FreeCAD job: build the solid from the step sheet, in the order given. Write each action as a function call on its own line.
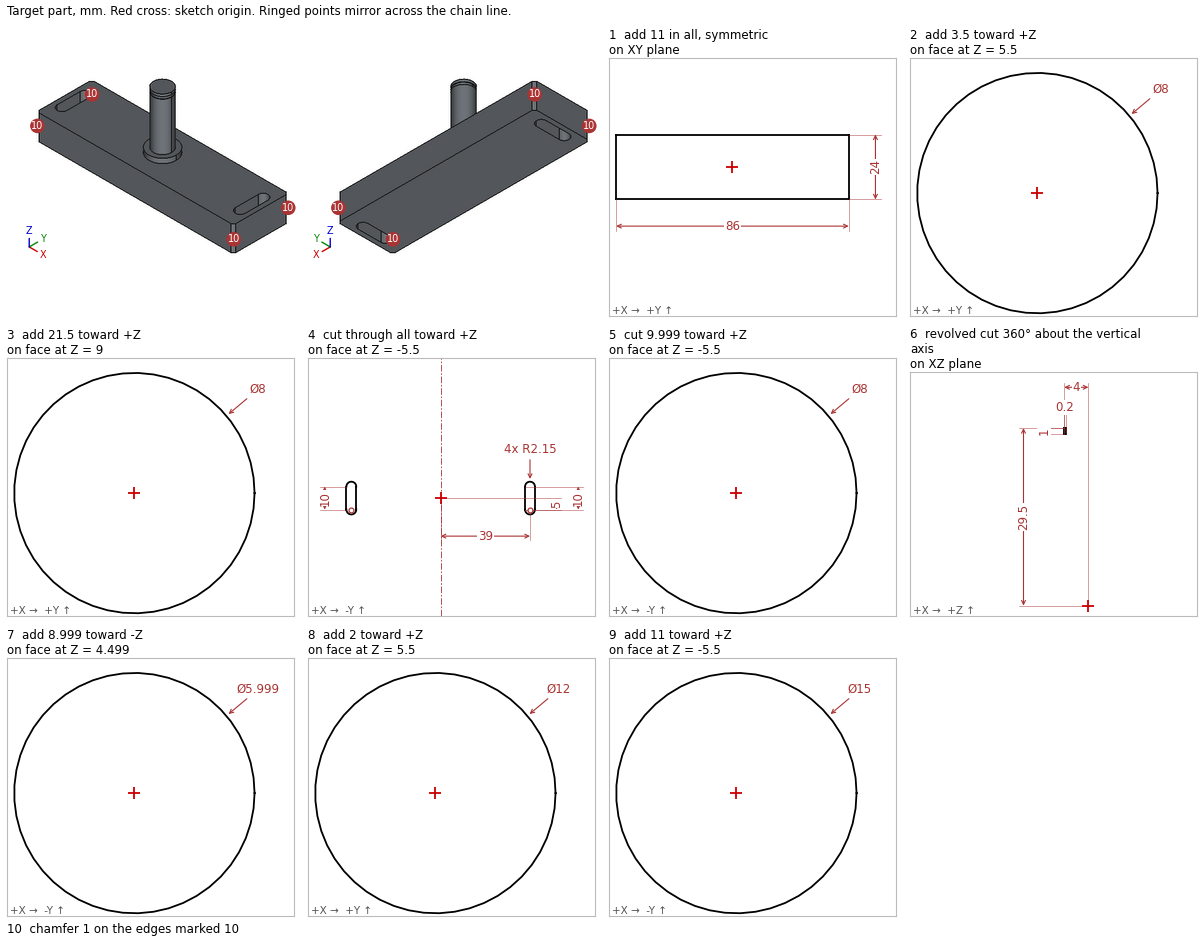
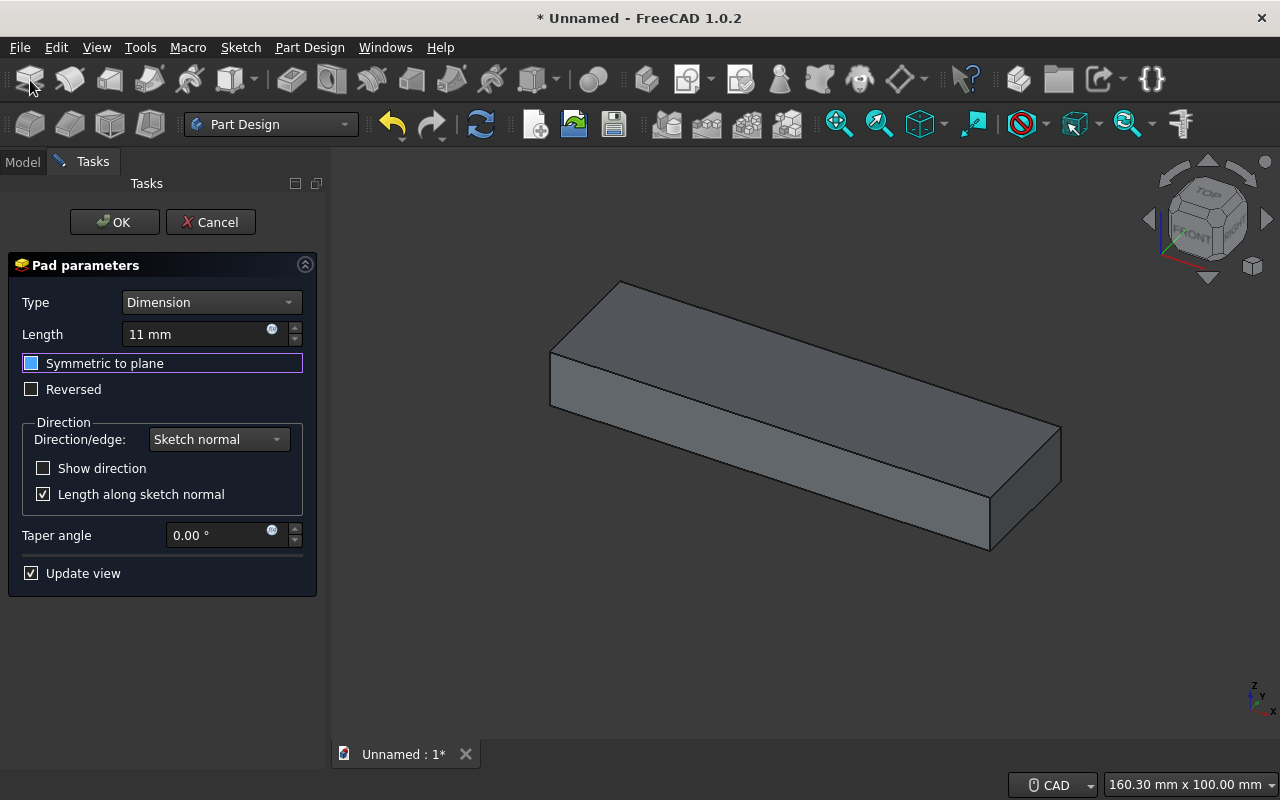
click(30, 363)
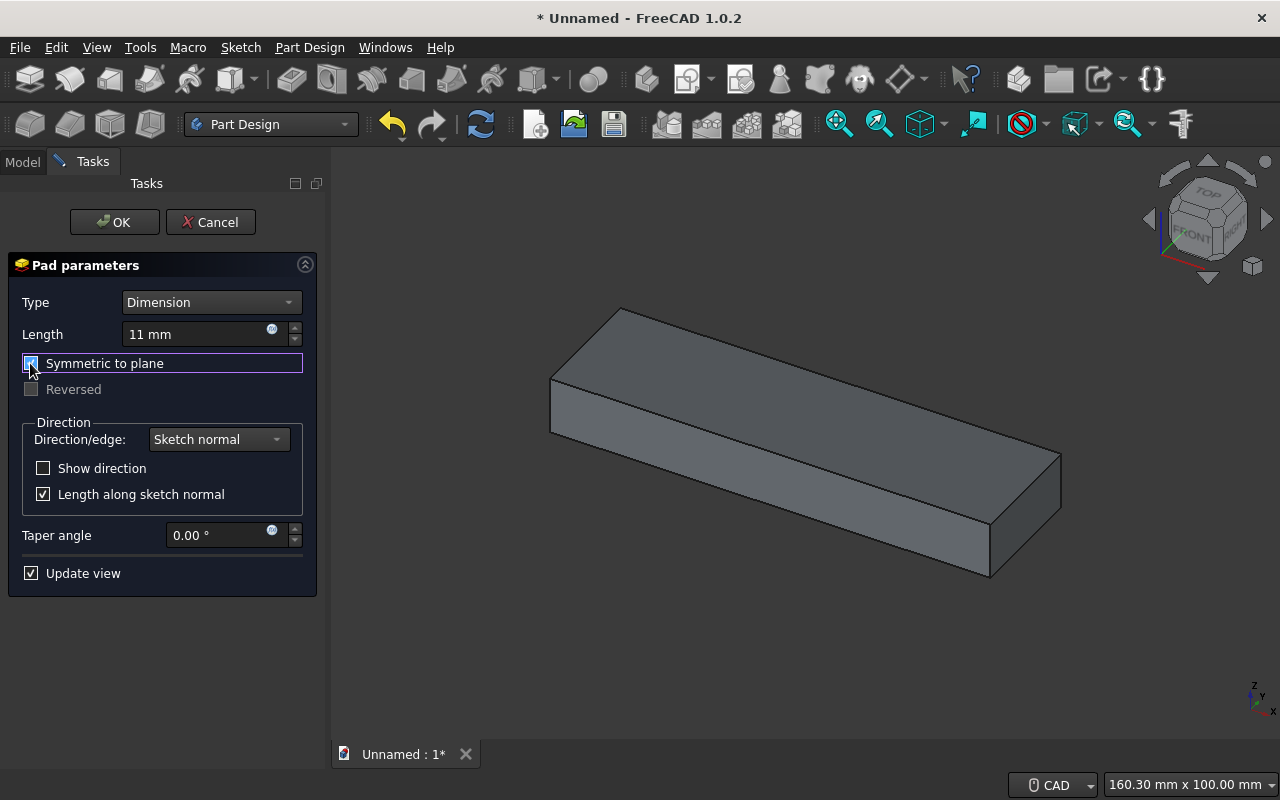
click(115, 222)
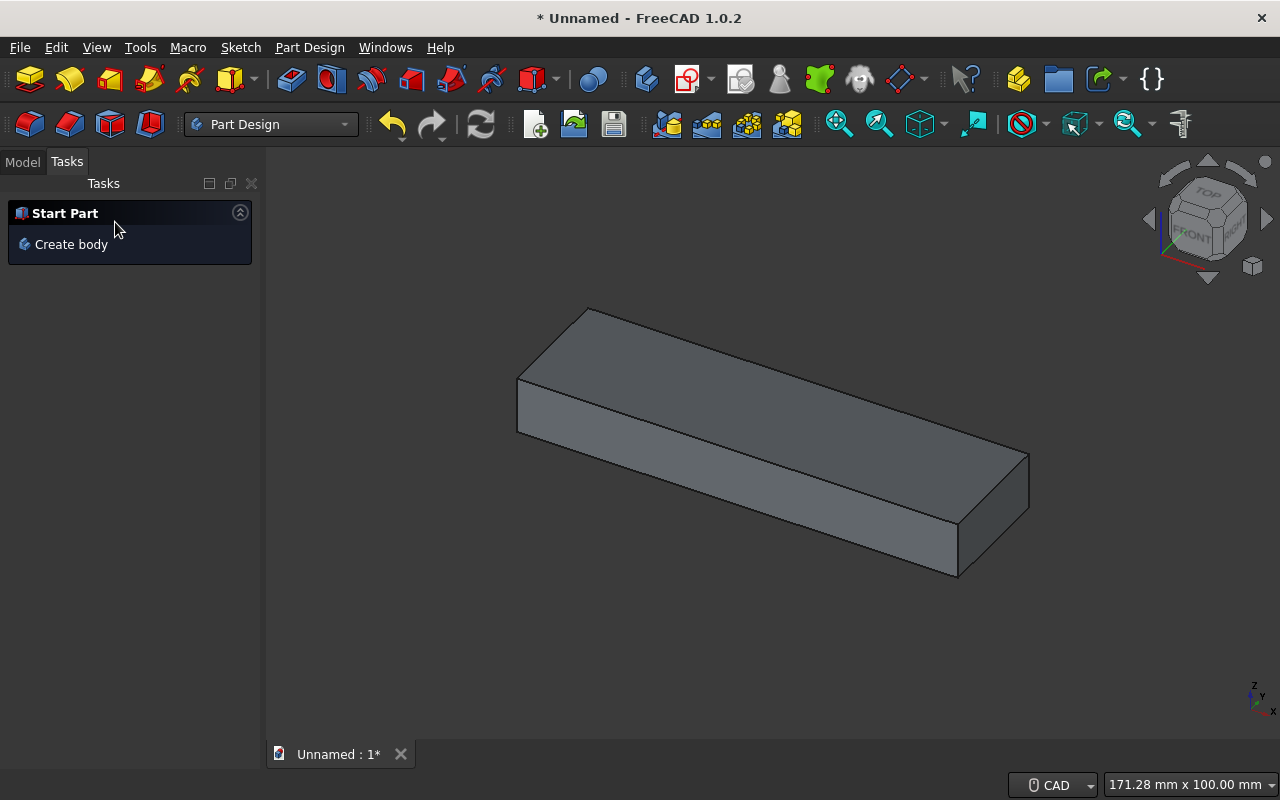
click(899, 457)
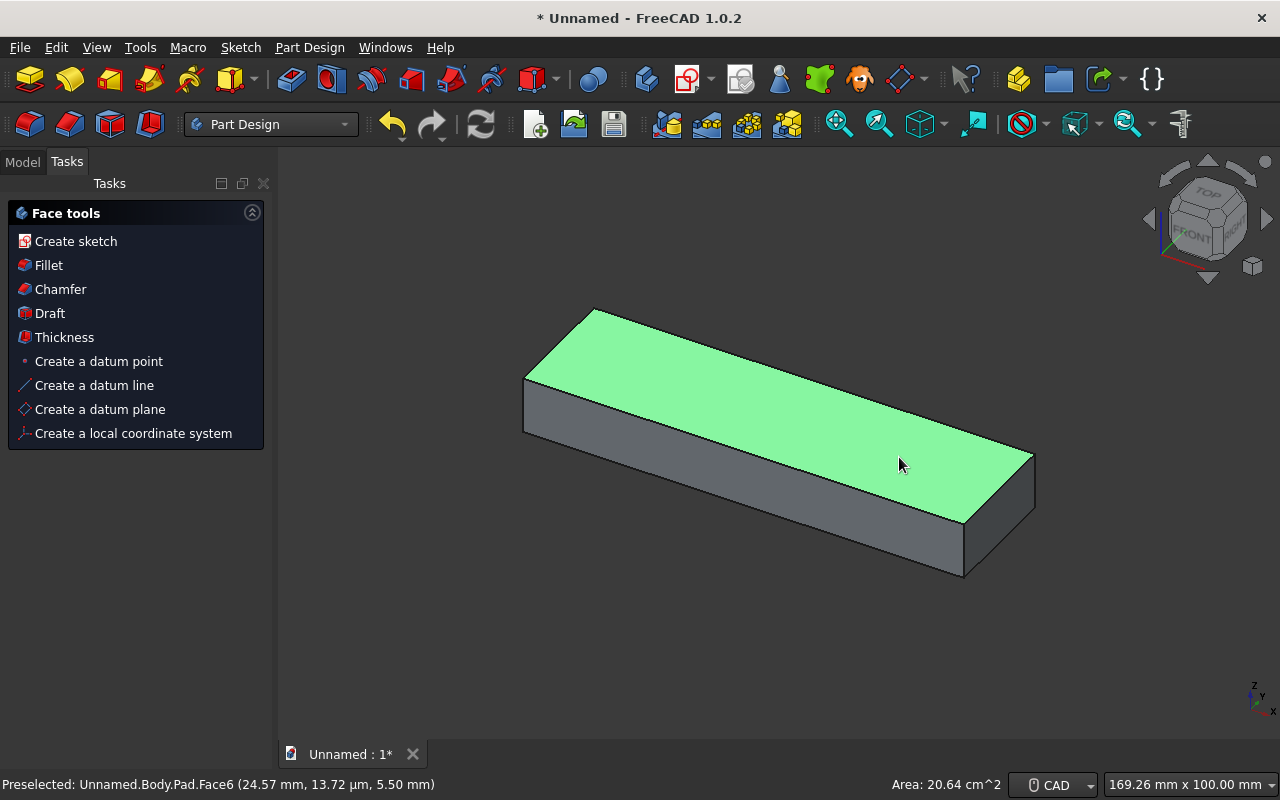
click(688, 80)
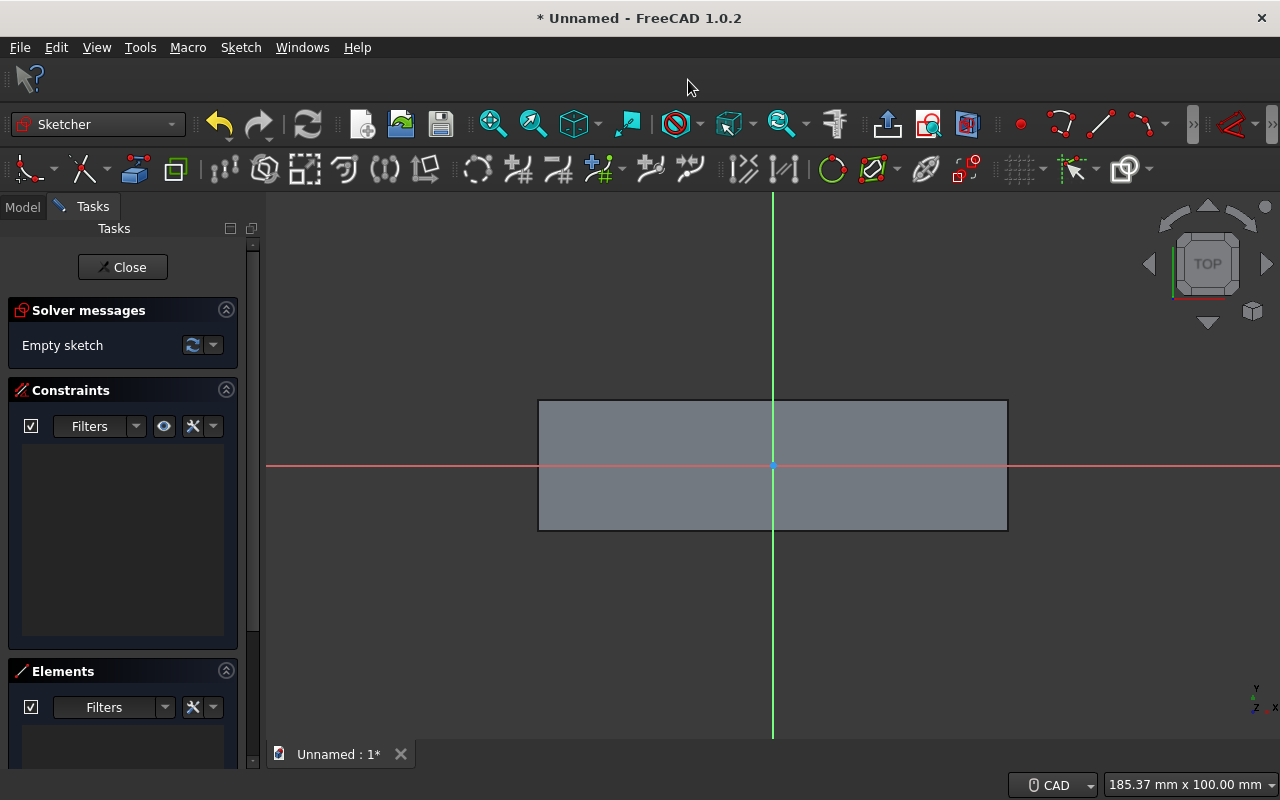
scroll(784, 466, up, 10)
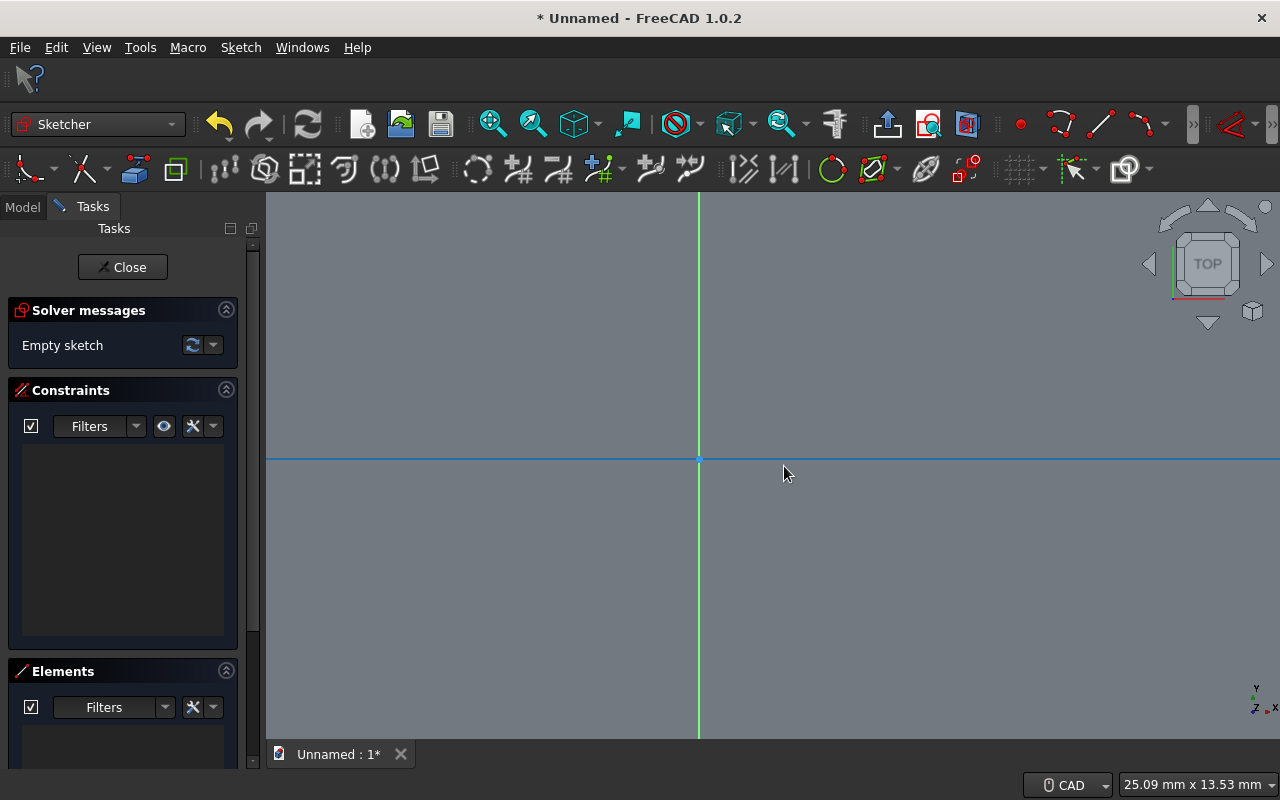
key(g)
key(c)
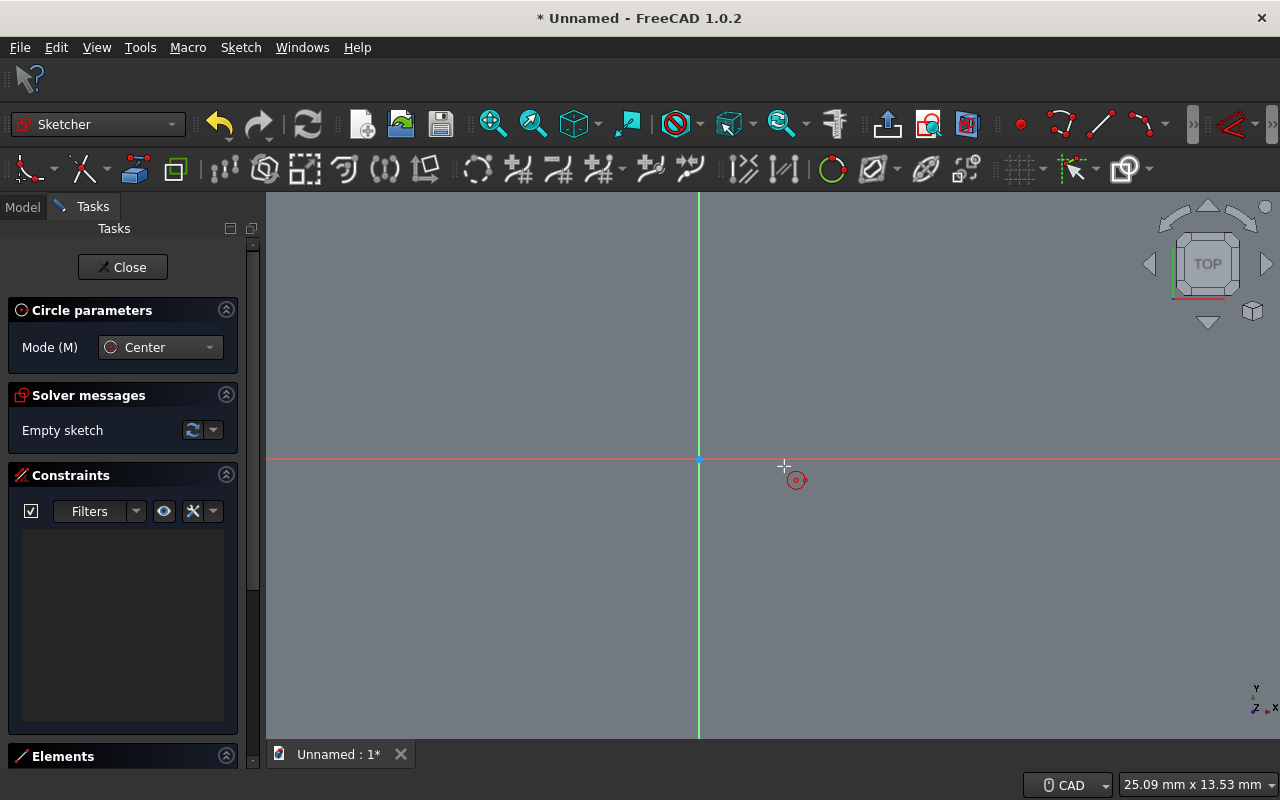
click(699, 459)
move(814, 345)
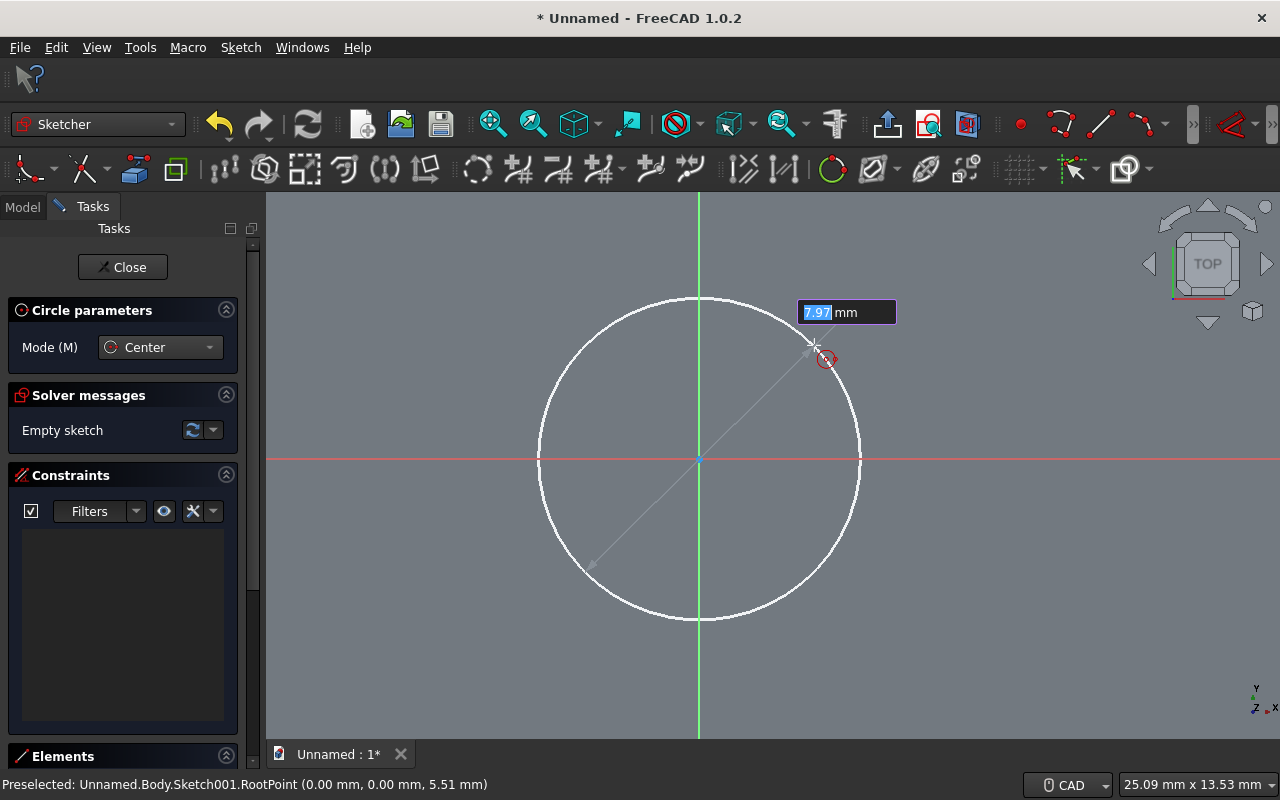
text(8)
key(Return)
key(Escape)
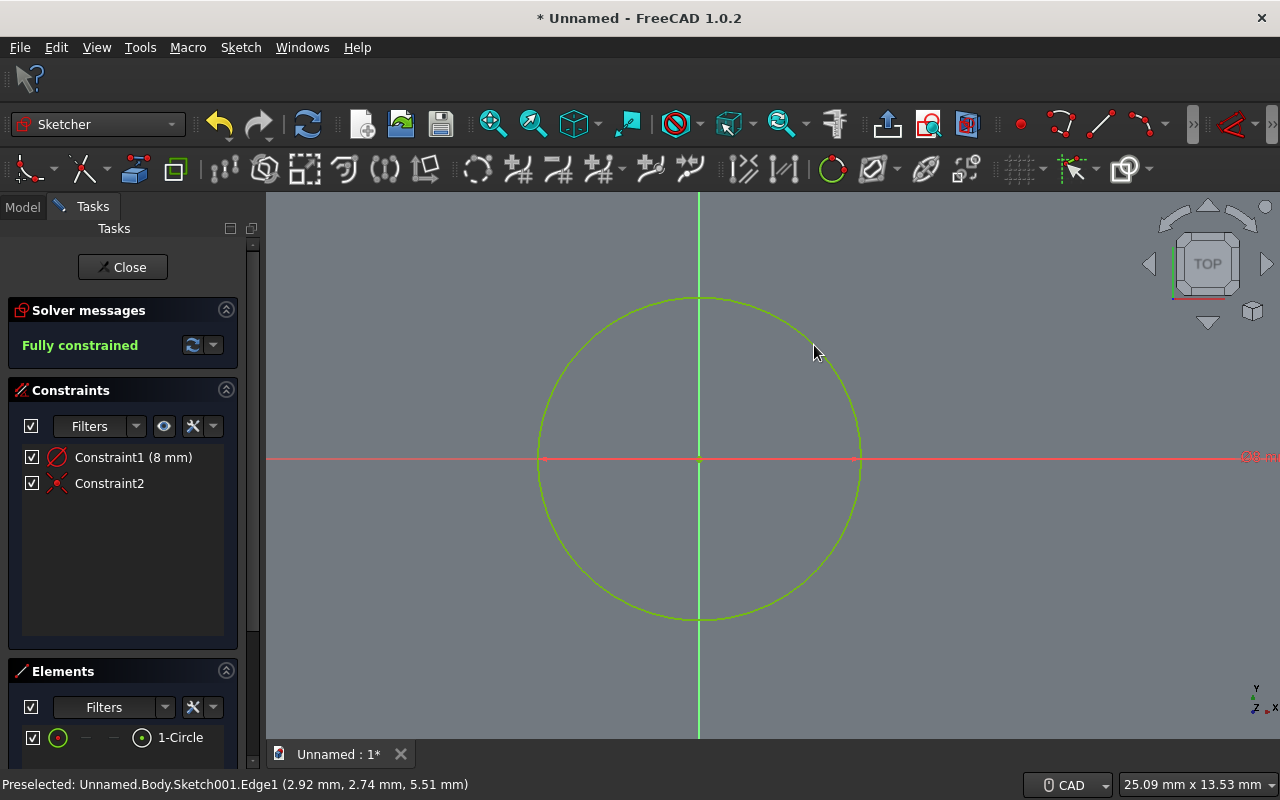
click(123, 267)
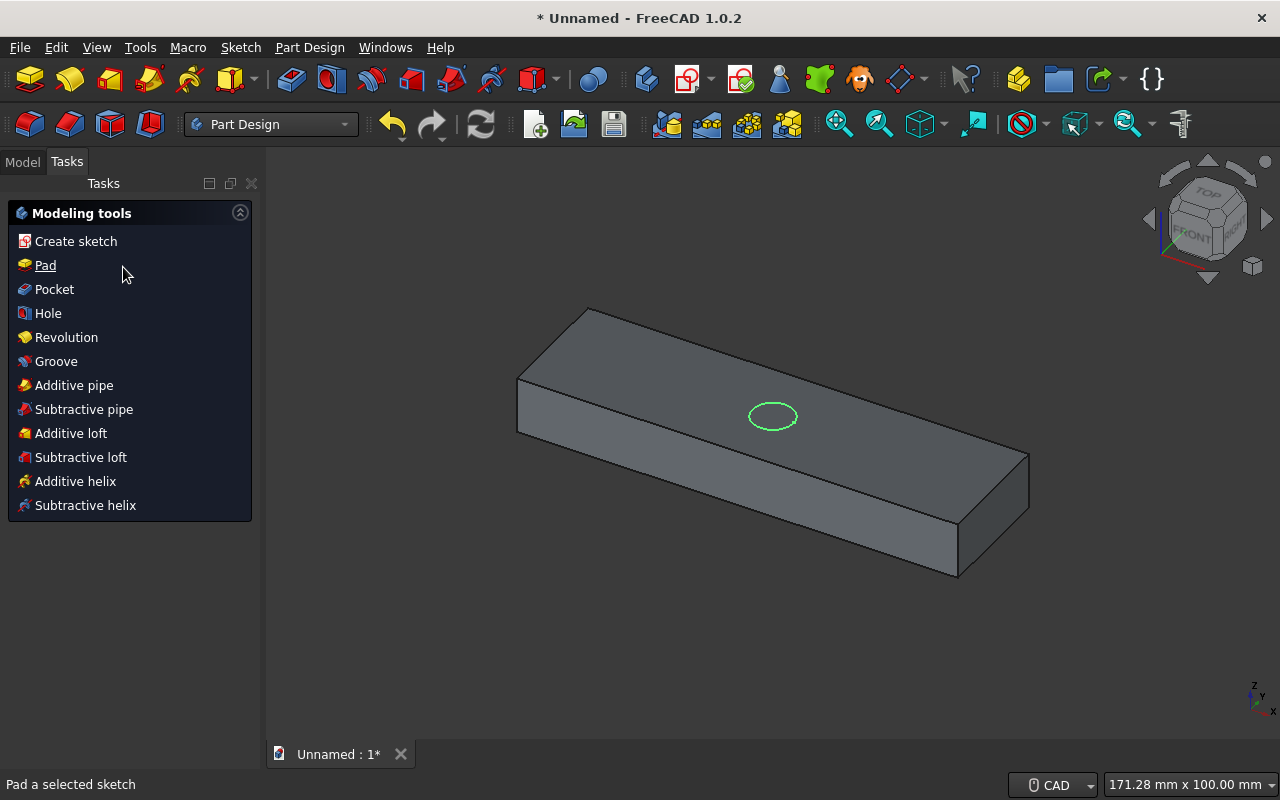
click(30, 80)